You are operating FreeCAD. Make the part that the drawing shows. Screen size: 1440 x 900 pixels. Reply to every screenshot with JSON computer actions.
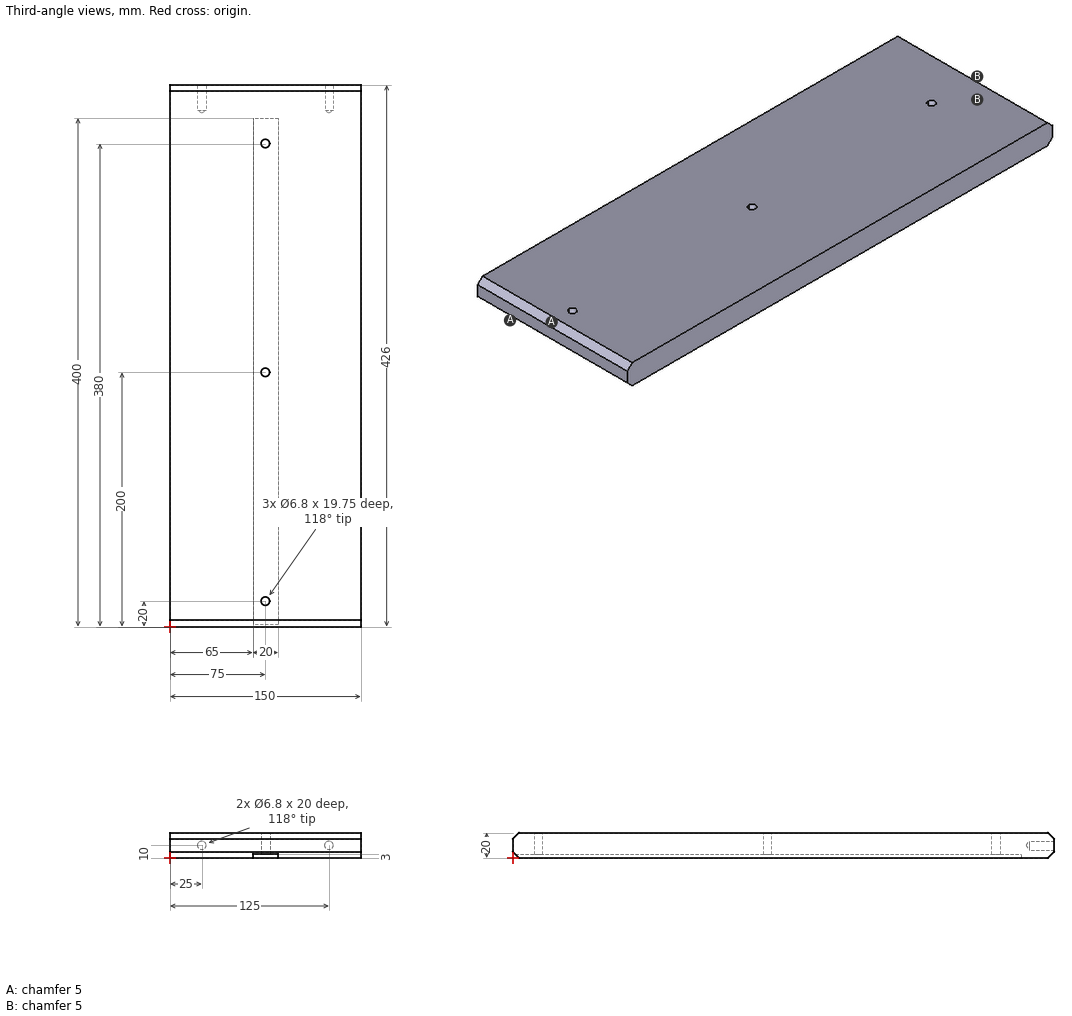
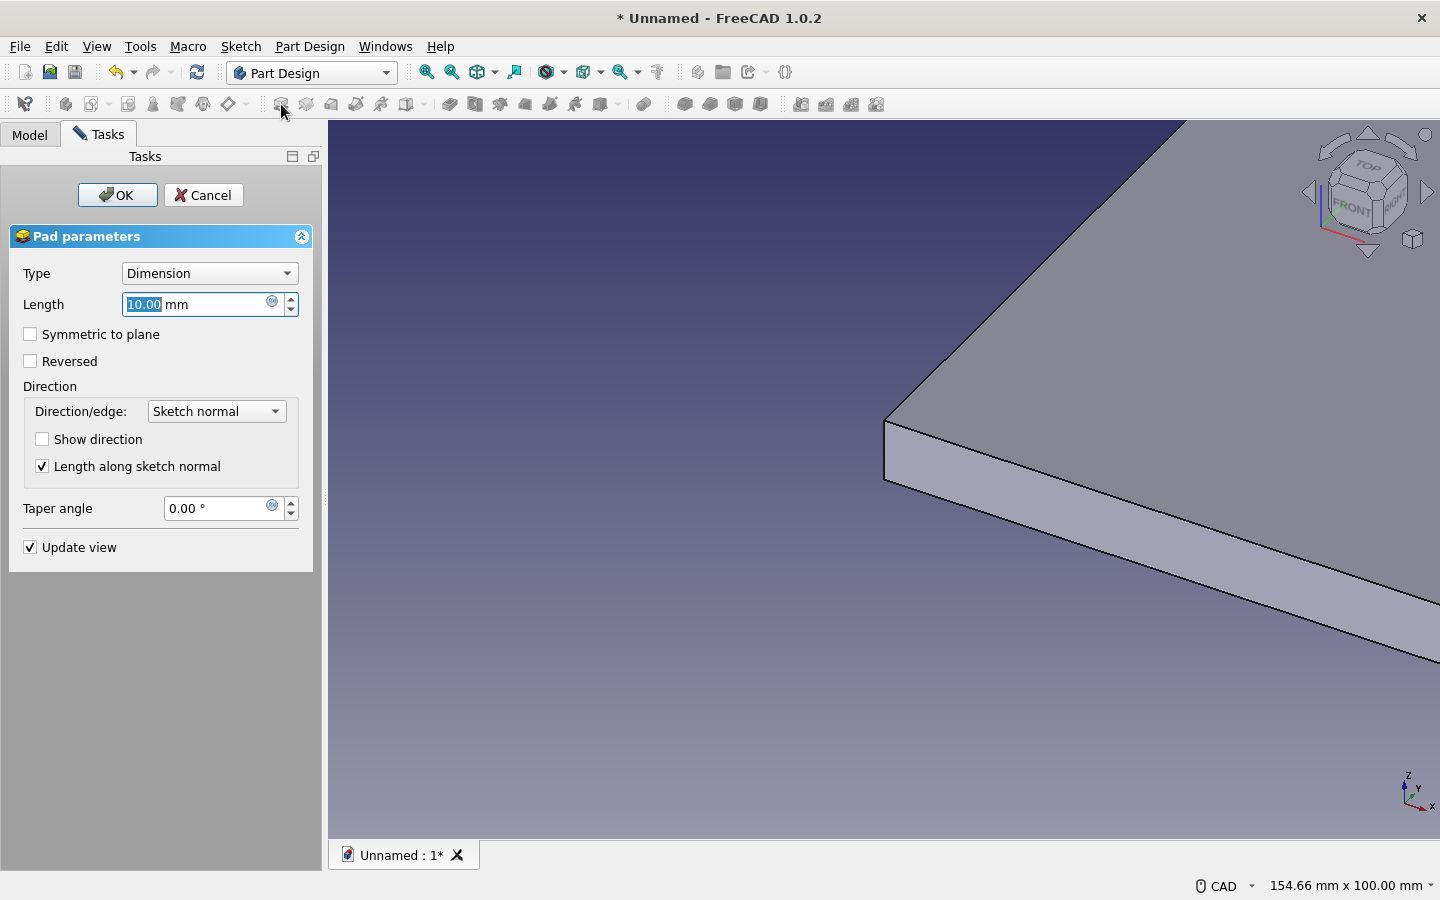
{"action": "type", "text": "20"}
{"action": "key", "text": "Tab"}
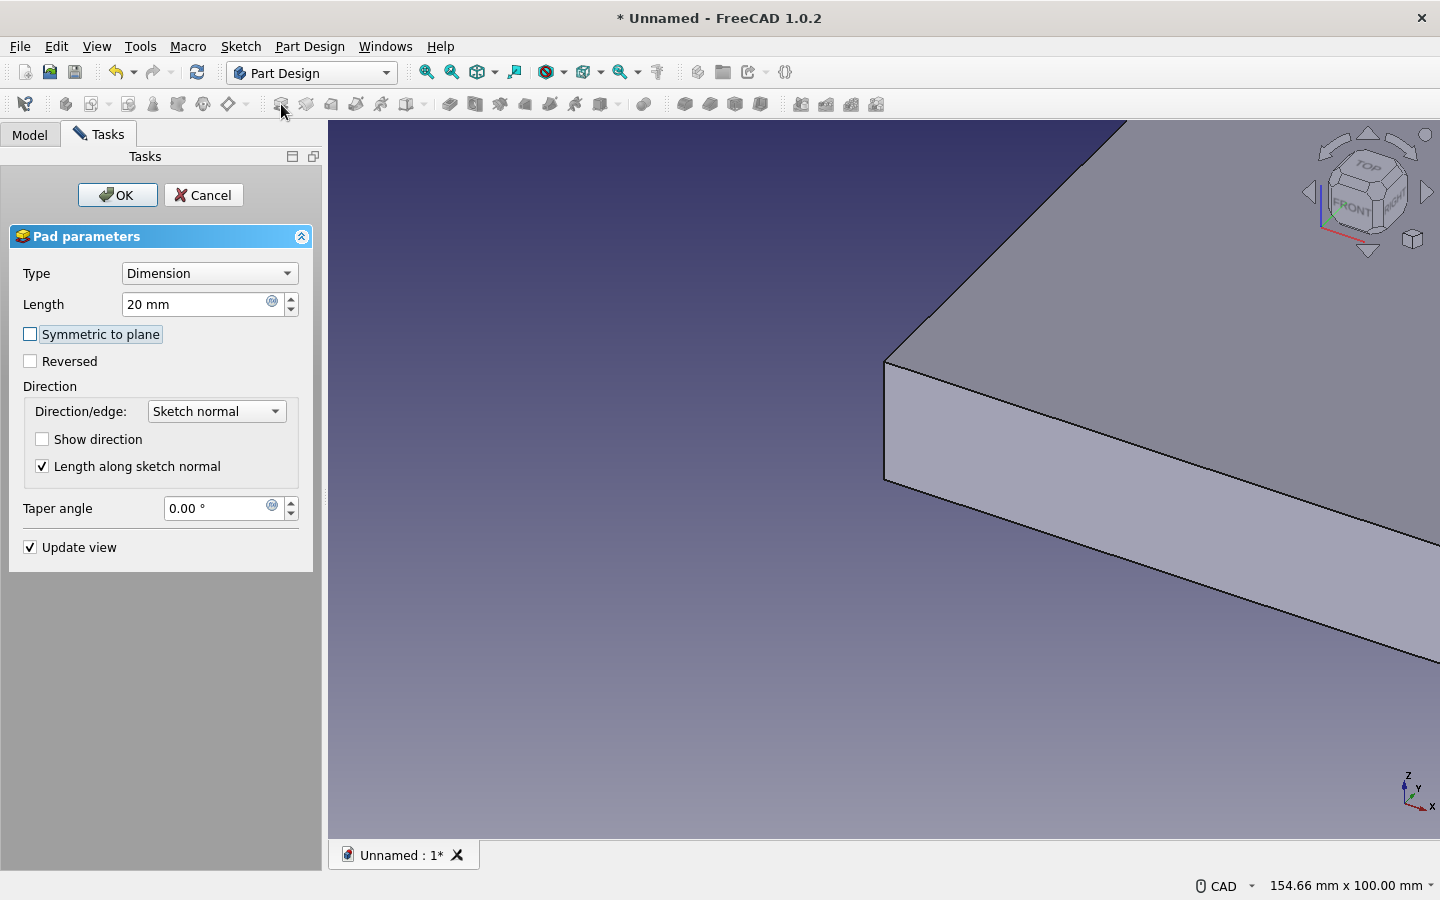
{"action": "left_click", "coordinate": [118, 195]}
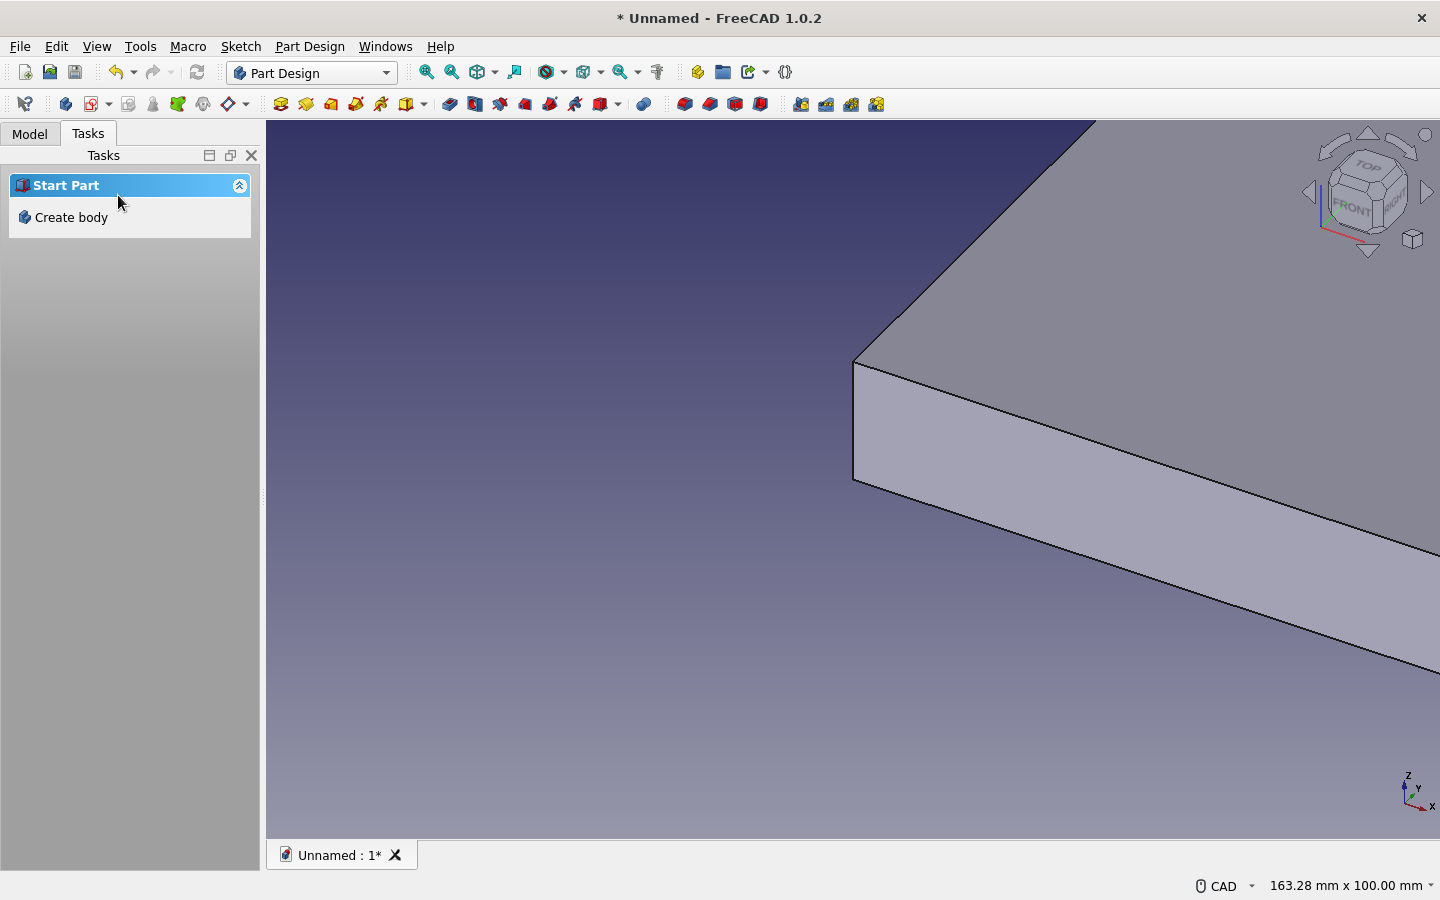
{"action": "left_click", "coordinate": [427, 72]}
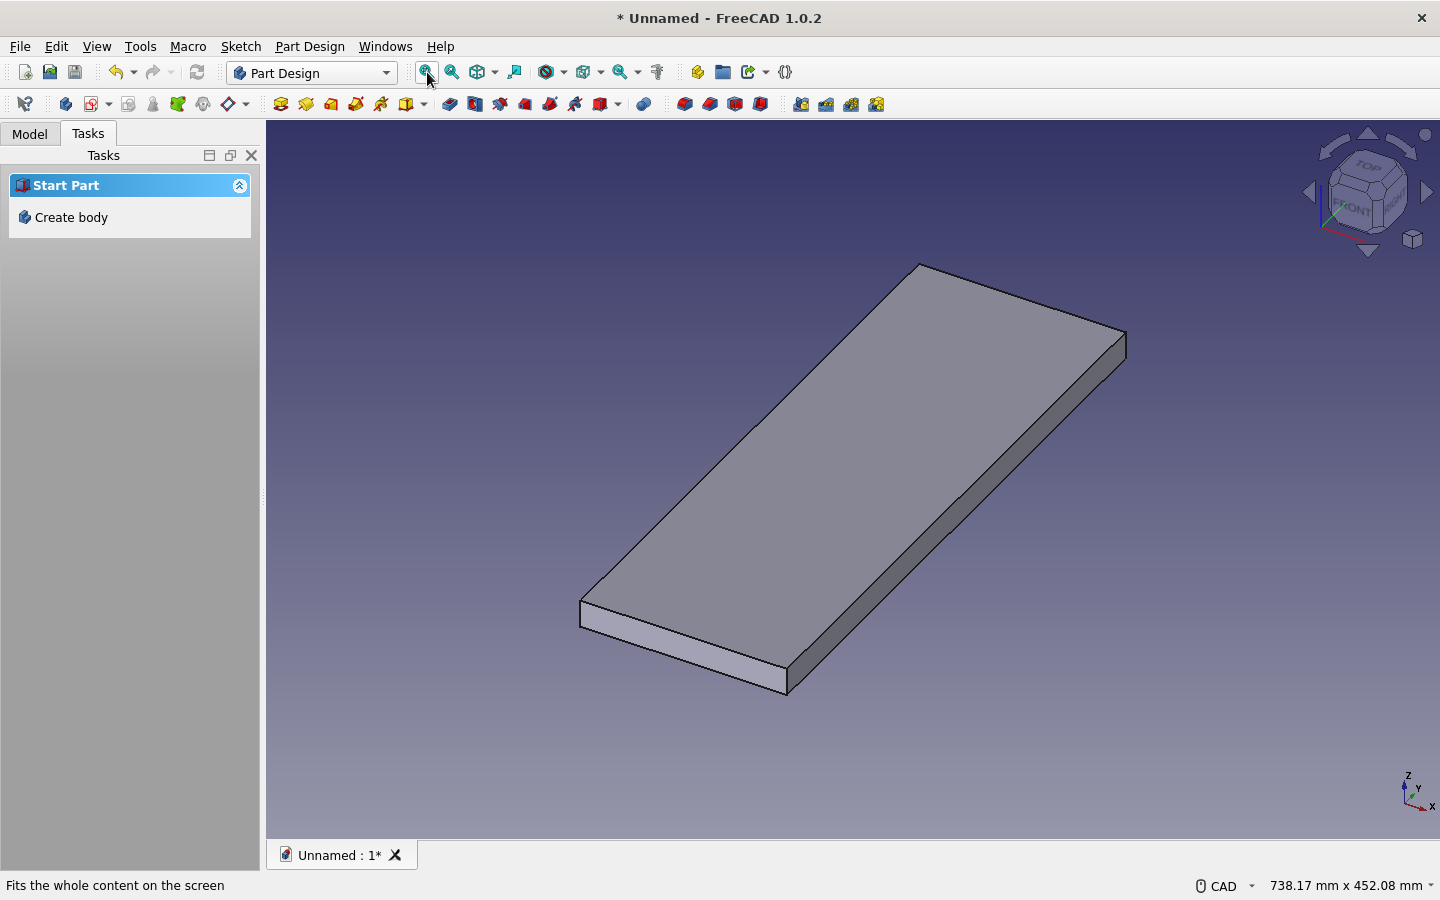
{"action": "left_click", "coordinate": [90, 104]}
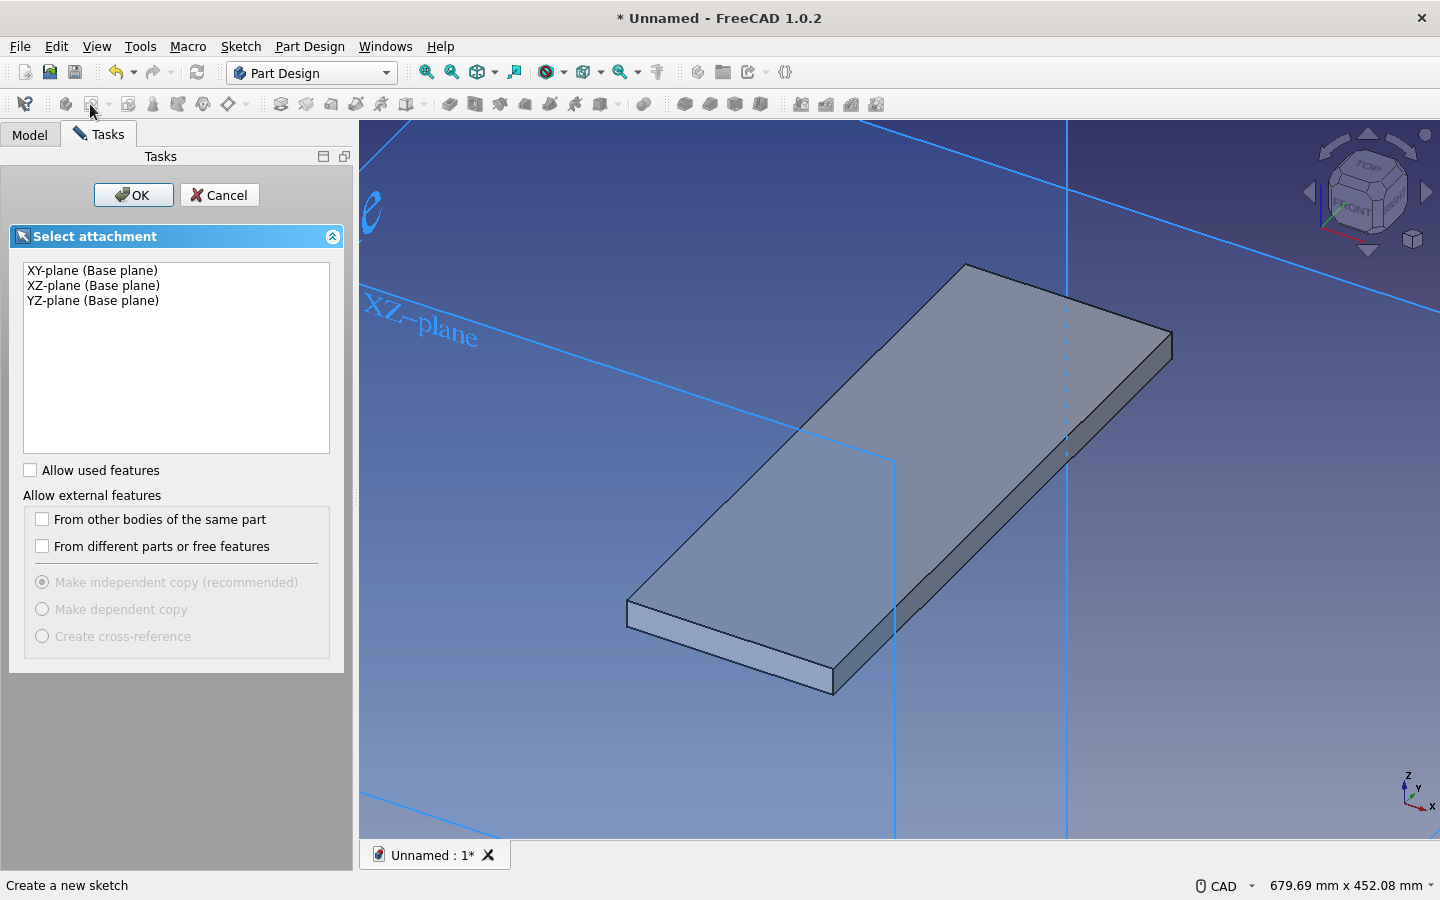
{"action": "left_click", "coordinate": [84, 270]}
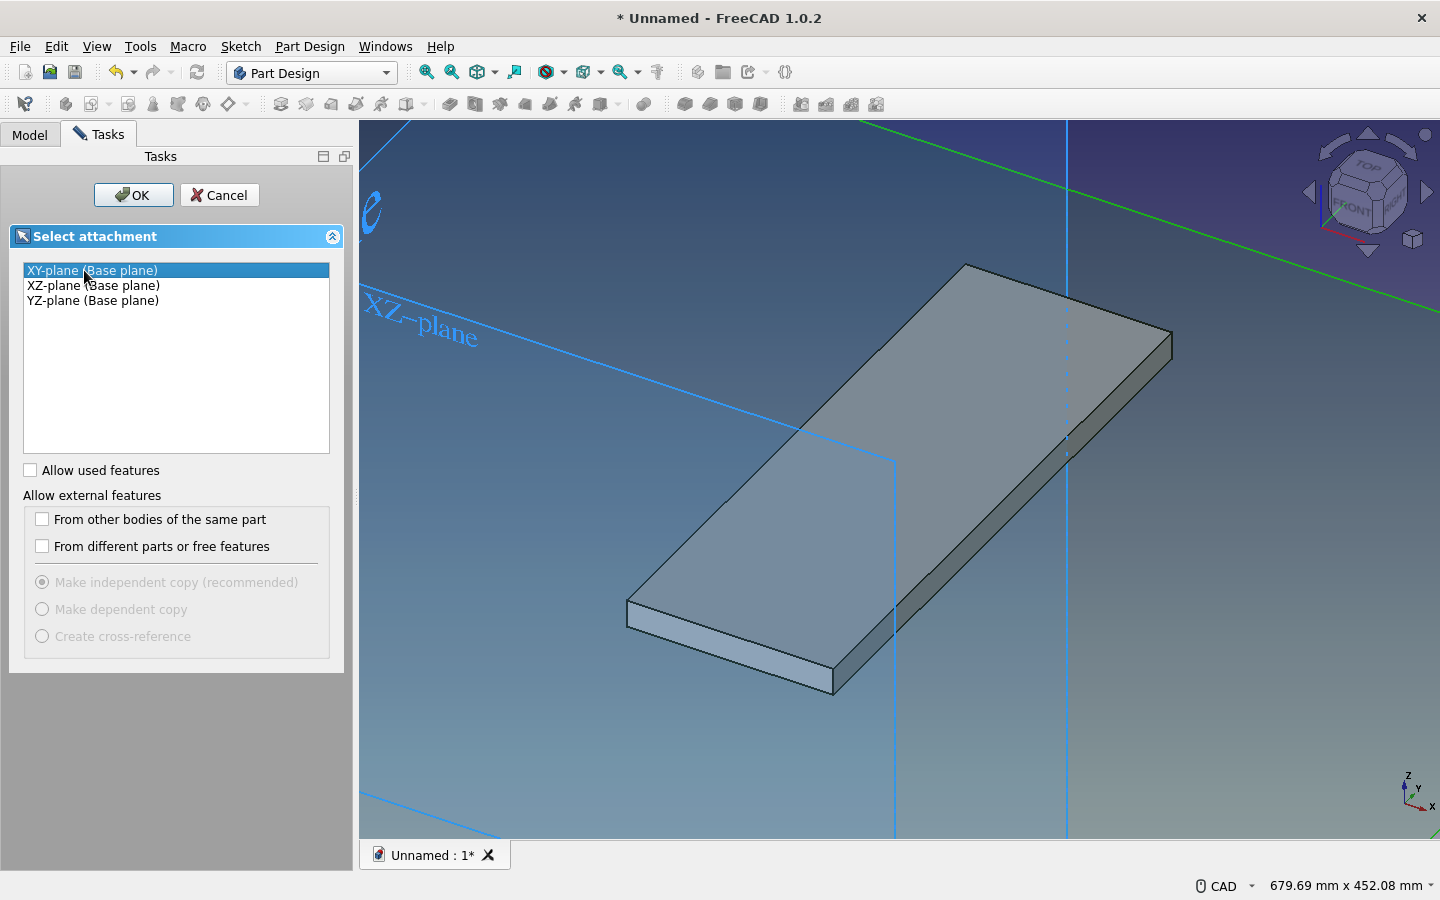
{"action": "left_click", "coordinate": [134, 195]}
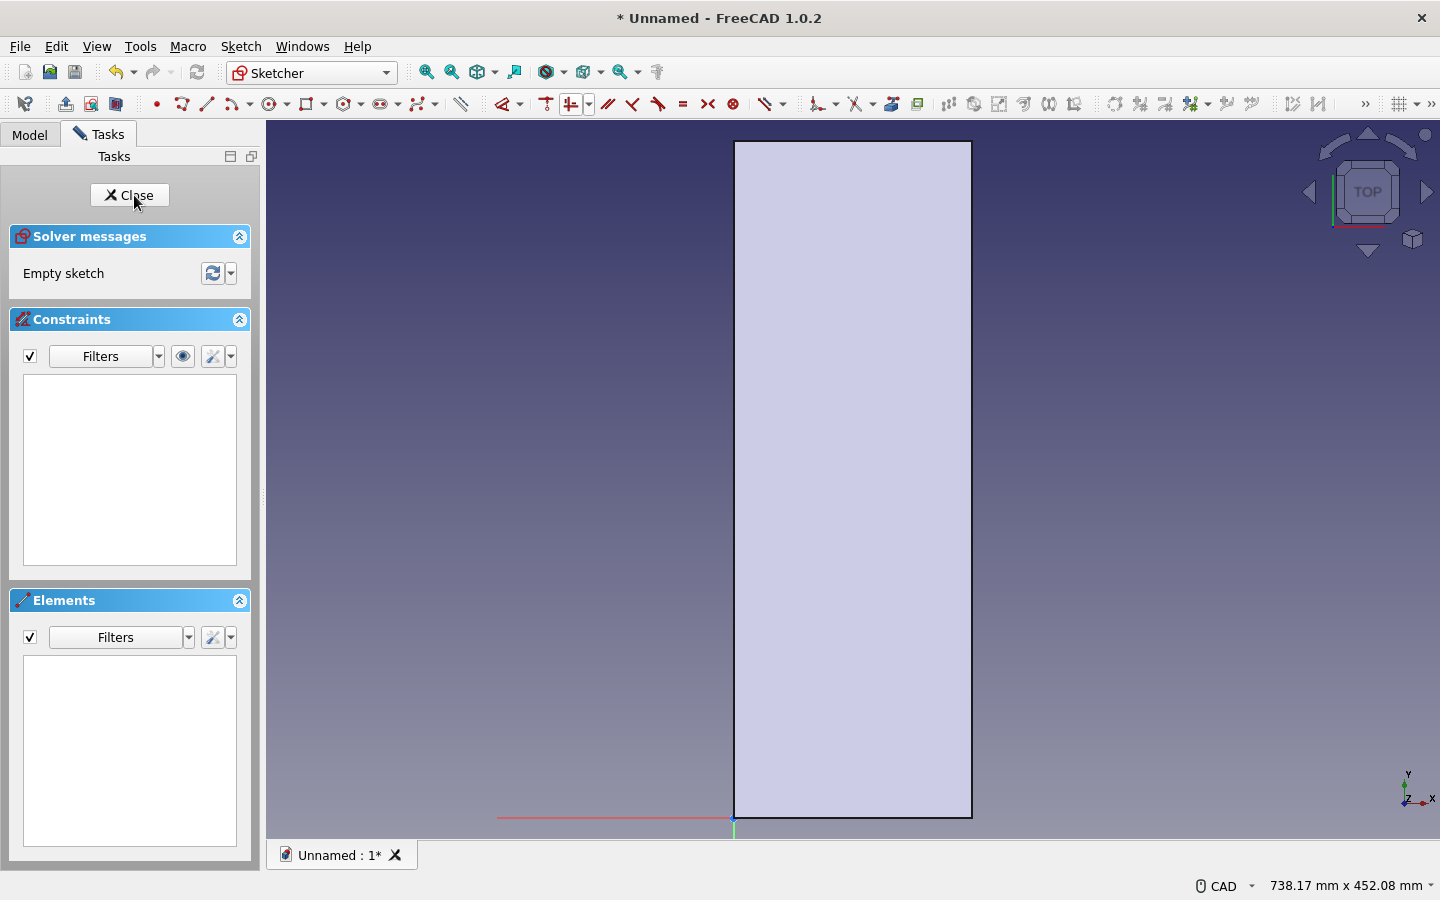
{"action": "left_click", "coordinate": [116, 104]}